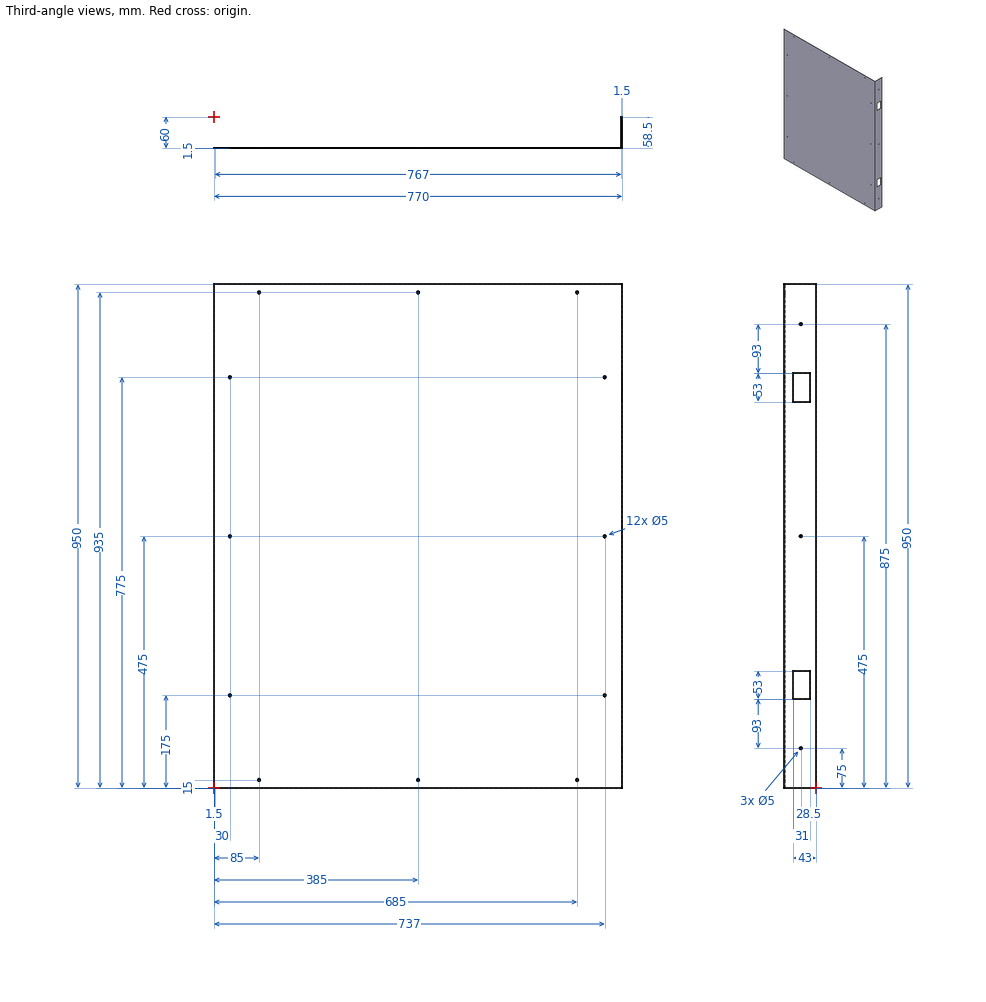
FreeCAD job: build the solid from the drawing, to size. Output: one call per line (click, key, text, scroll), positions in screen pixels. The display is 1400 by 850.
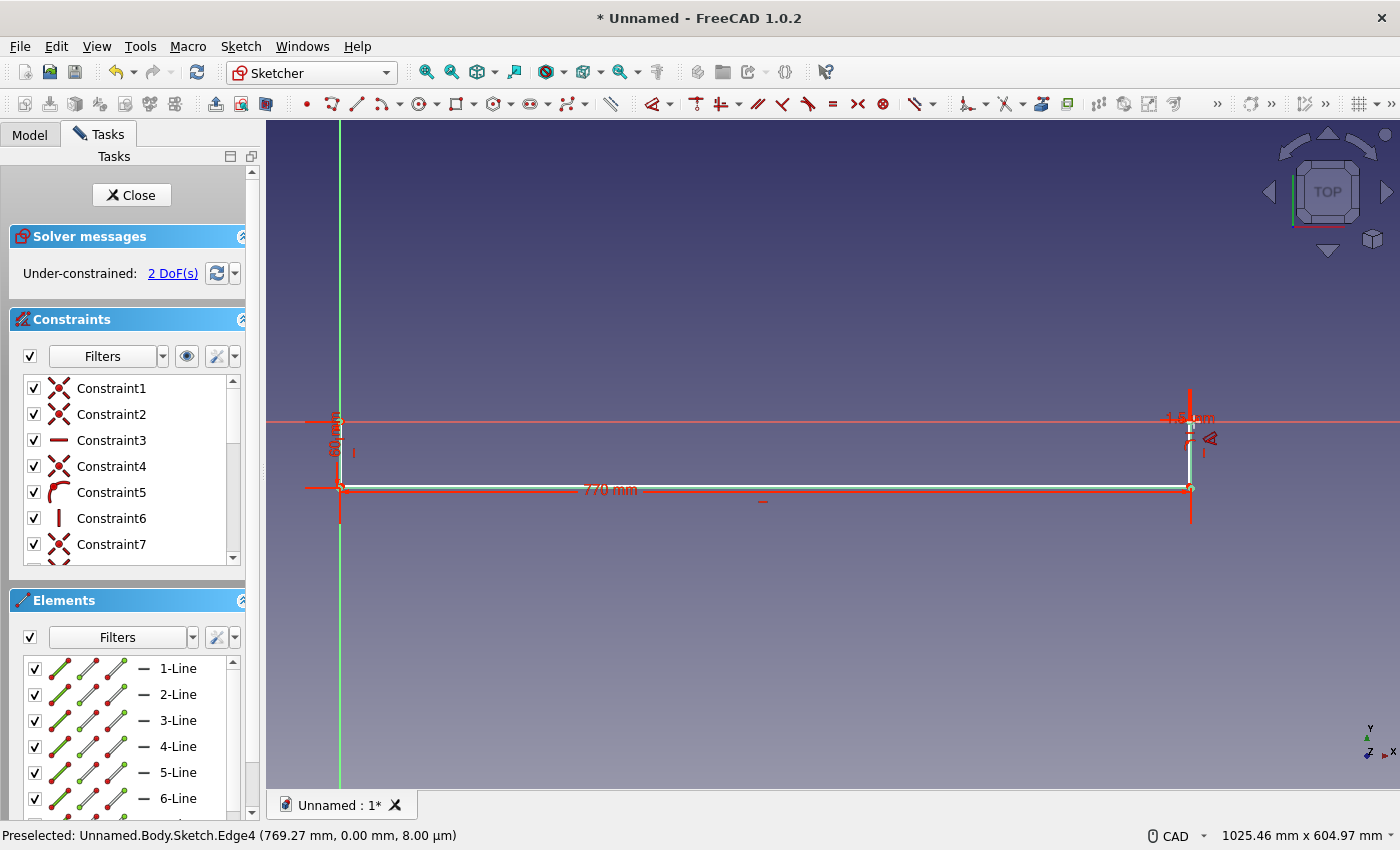
scroll(935, 486, up, 11)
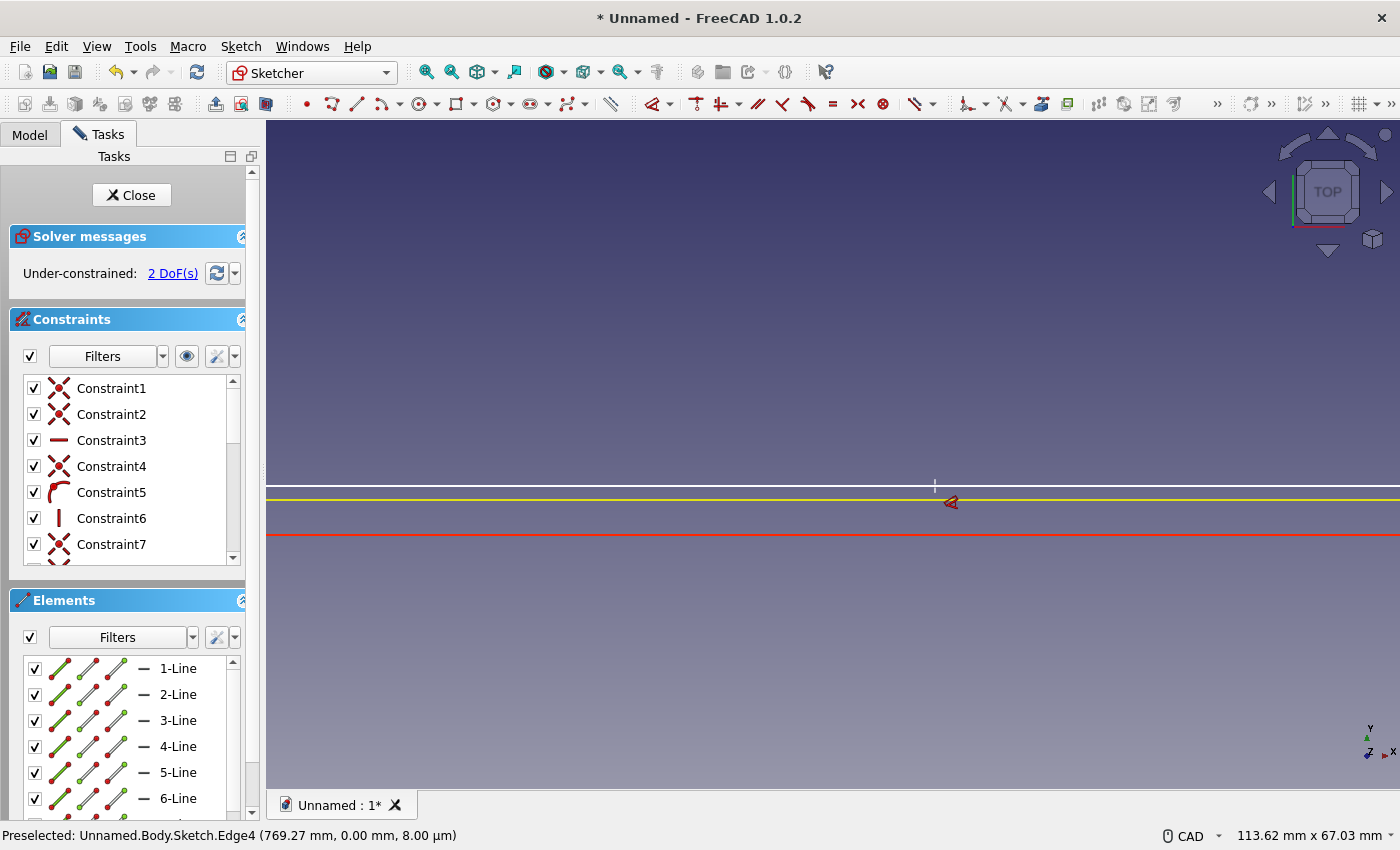
click(931, 486)
click(764, 520)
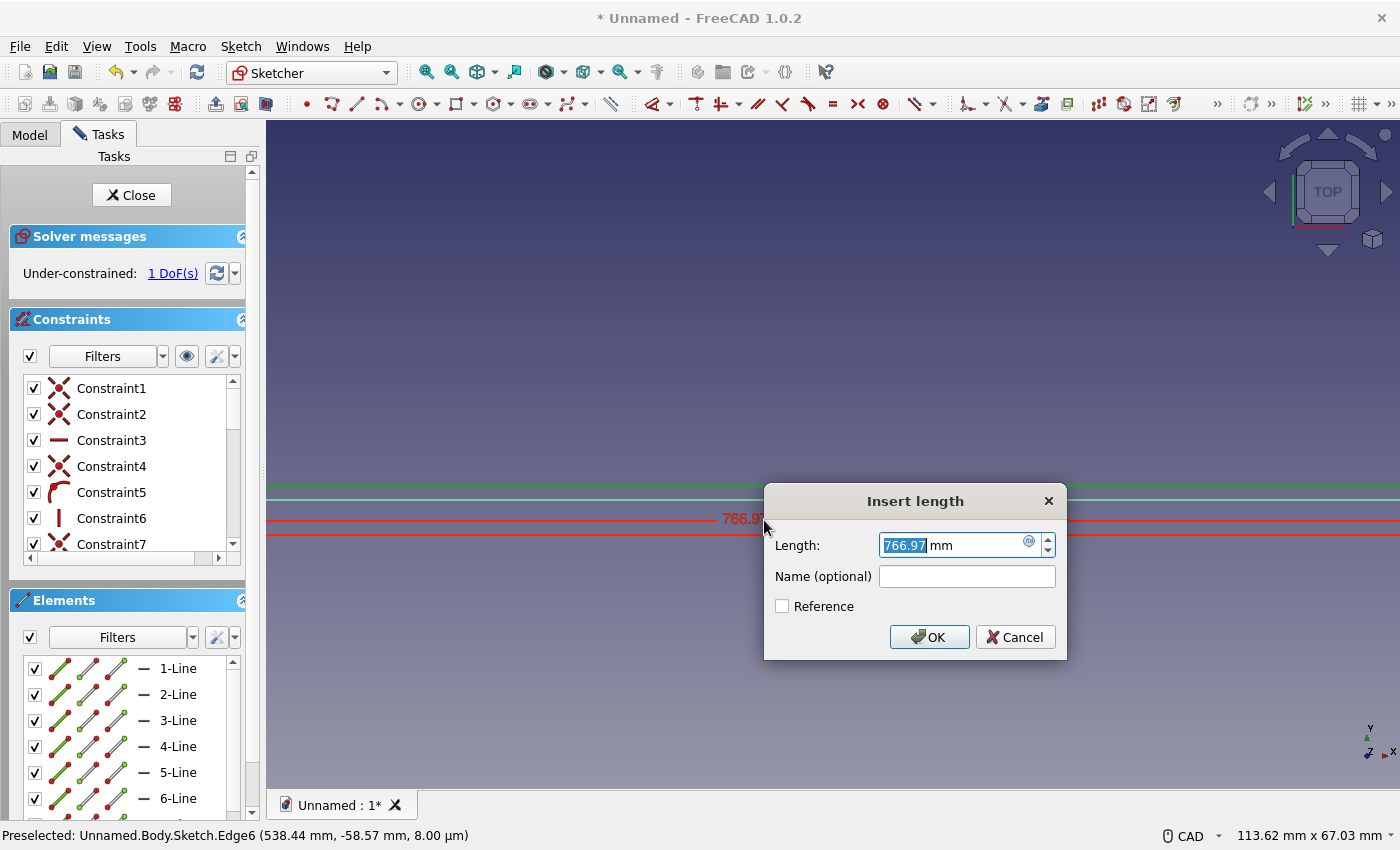
text(767)
key(Return)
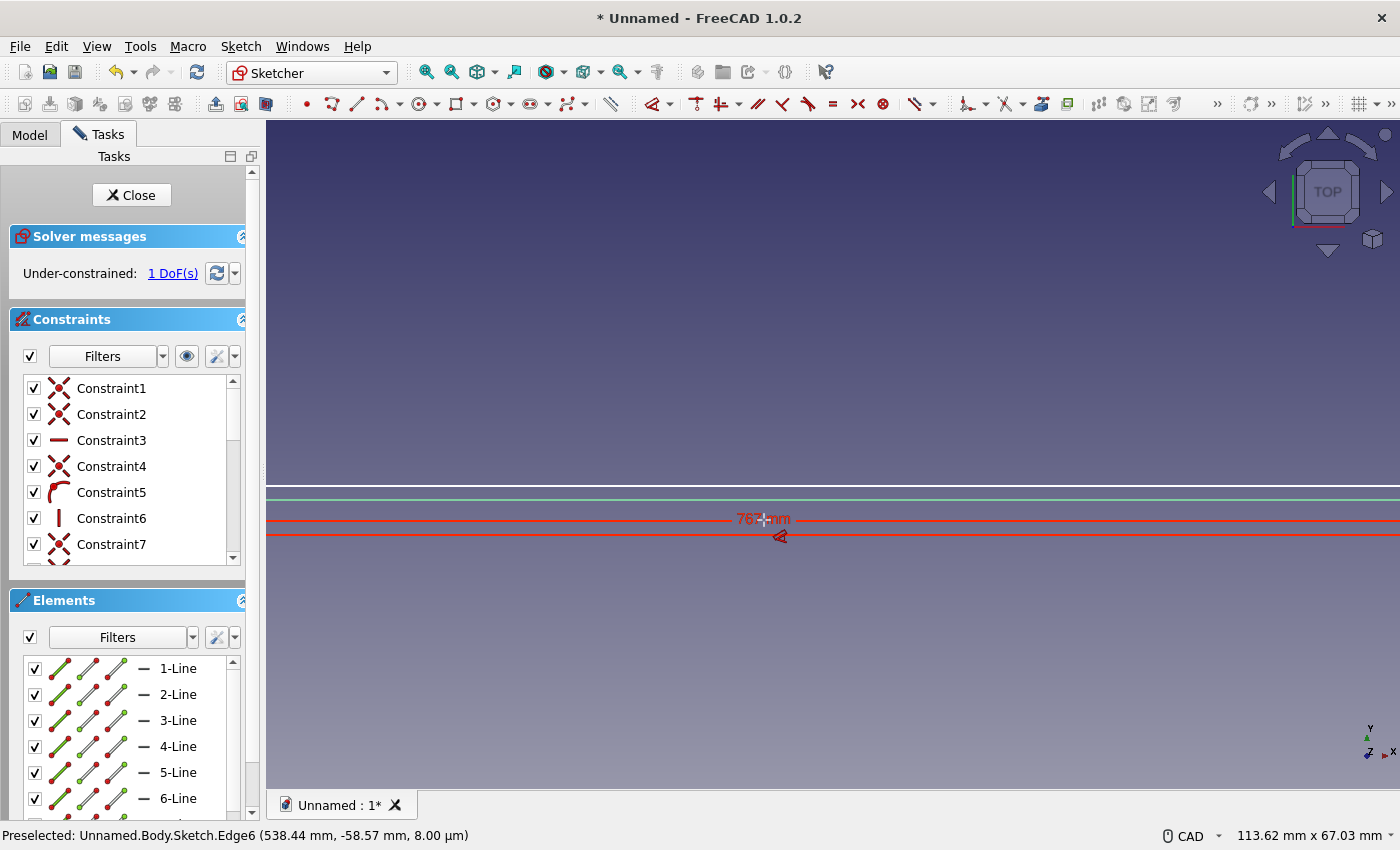
scroll(901, 480, down, 12)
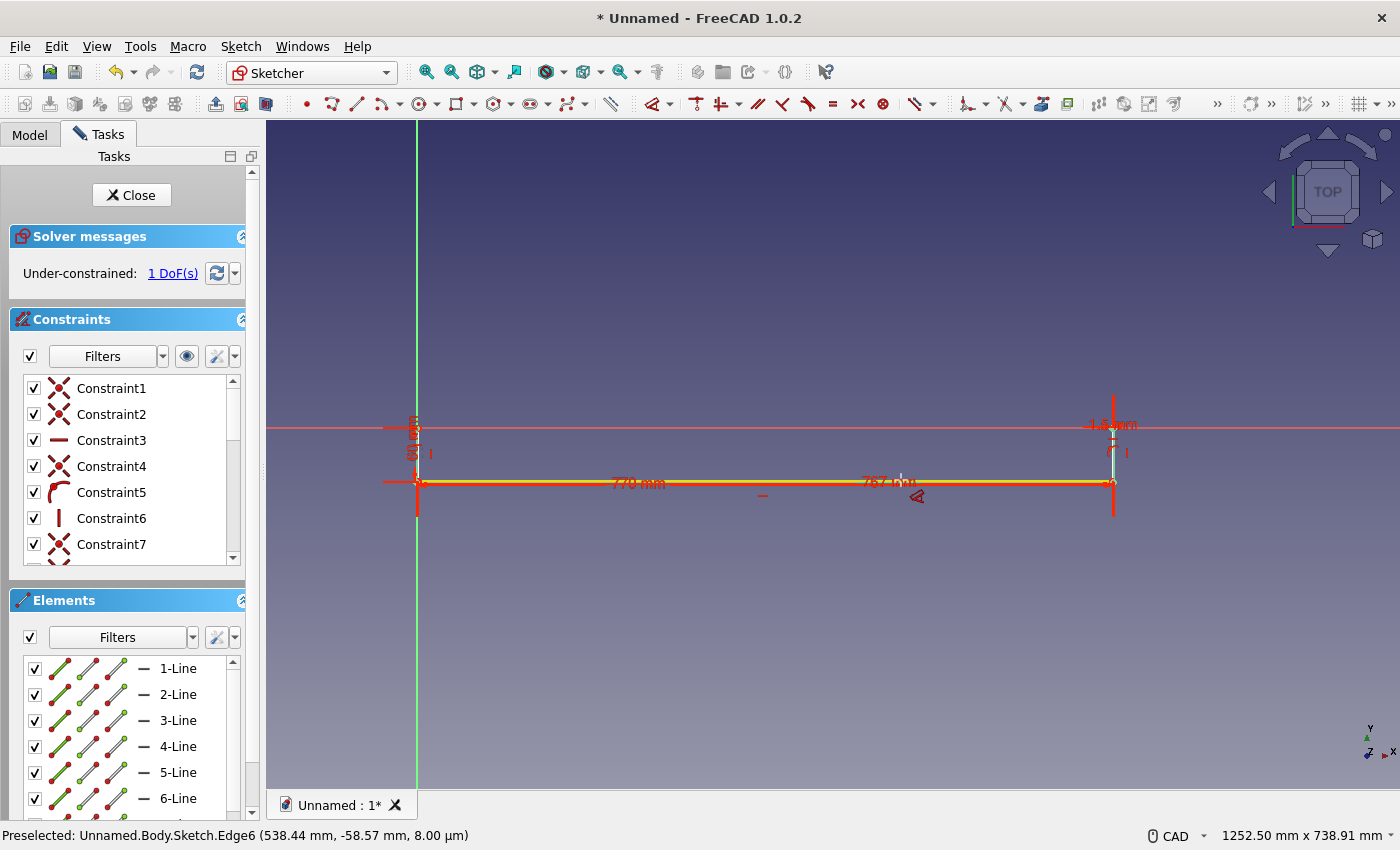
scroll(1113, 444, up, 12)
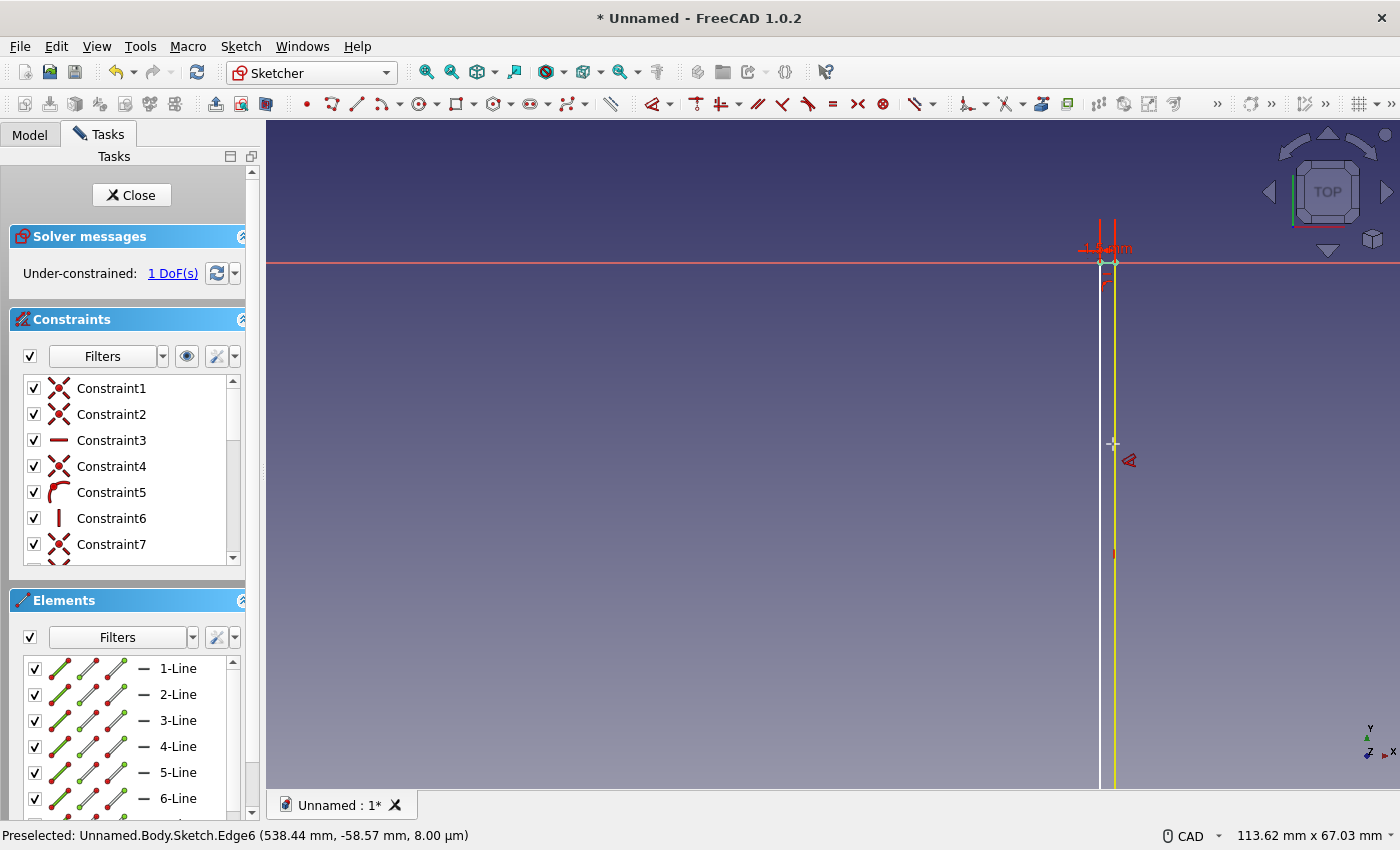
click(1100, 438)
click(1134, 512)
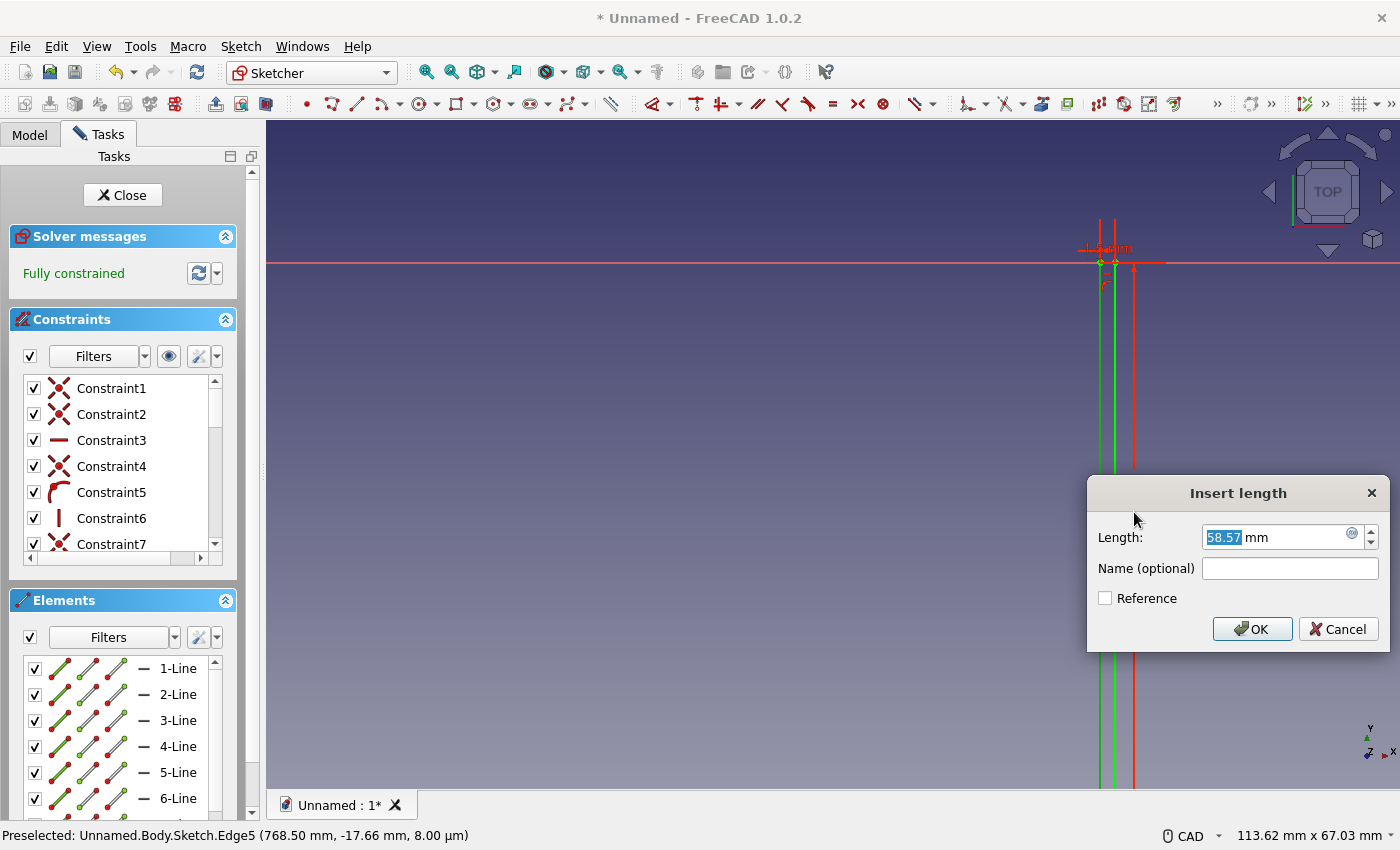
text(58.5)
key(Return)
key(Escape)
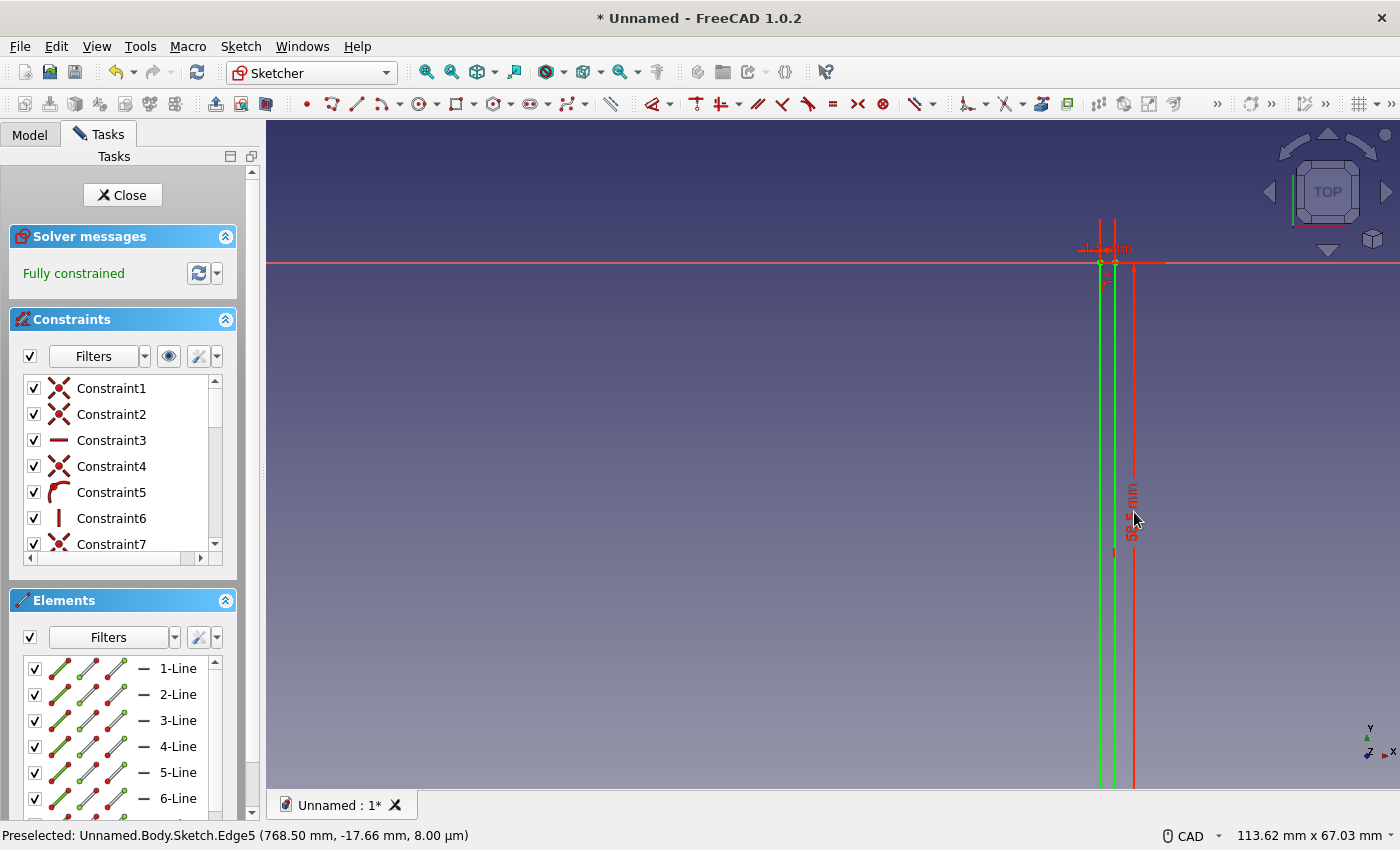
click(123, 195)